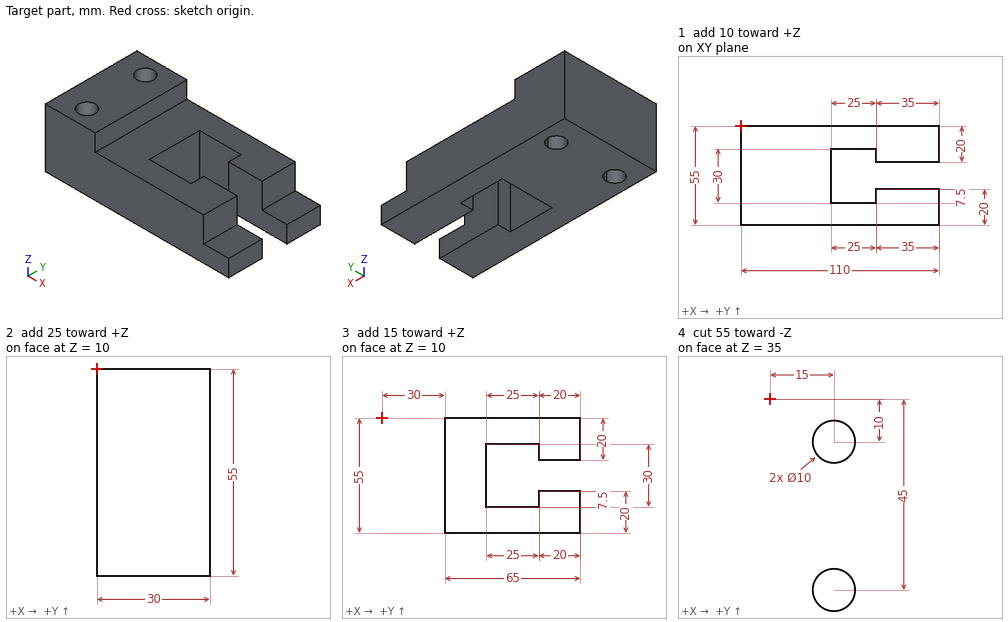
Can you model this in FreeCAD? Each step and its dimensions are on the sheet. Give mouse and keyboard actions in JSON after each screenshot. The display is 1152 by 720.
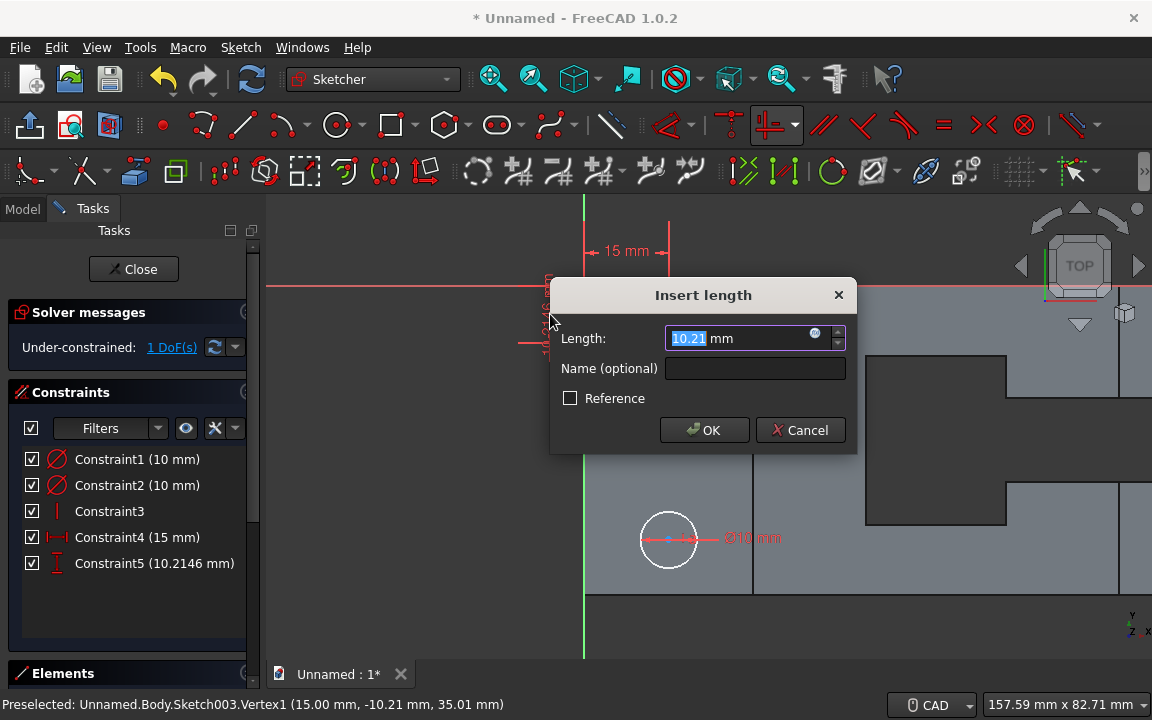
{"action": "type", "text": "10"}
{"action": "key", "text": "Return"}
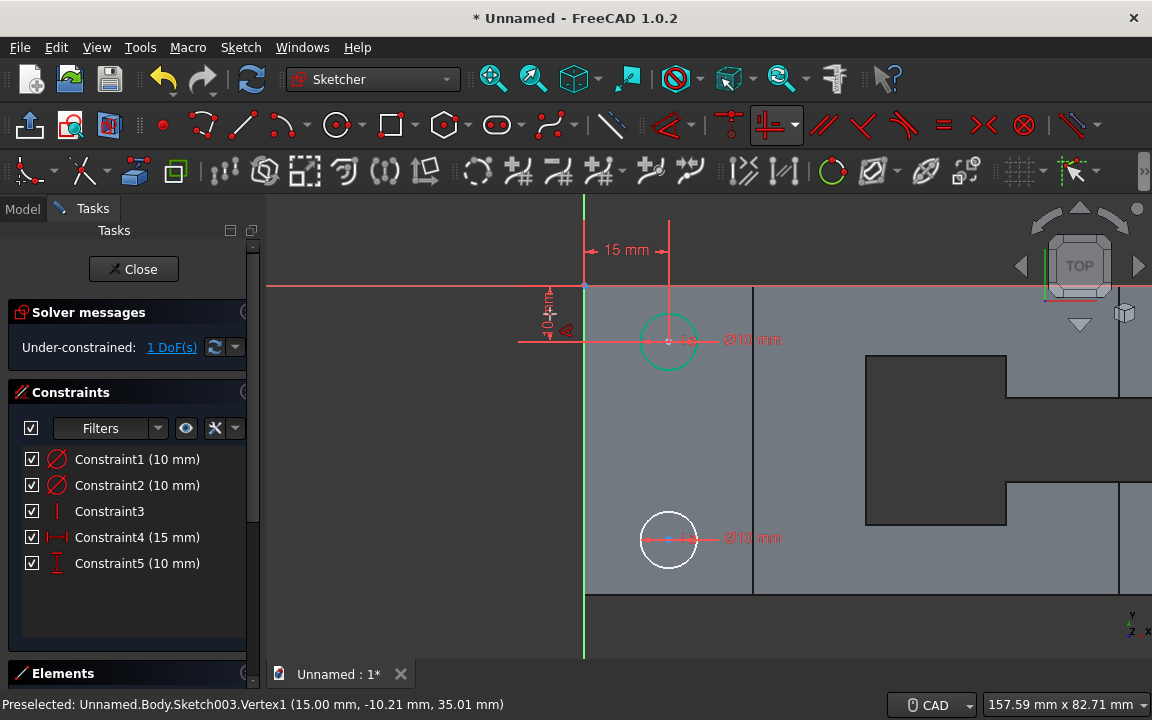
{"action": "left_click", "coordinate": [669, 540]}
{"action": "left_click", "coordinate": [550, 413]}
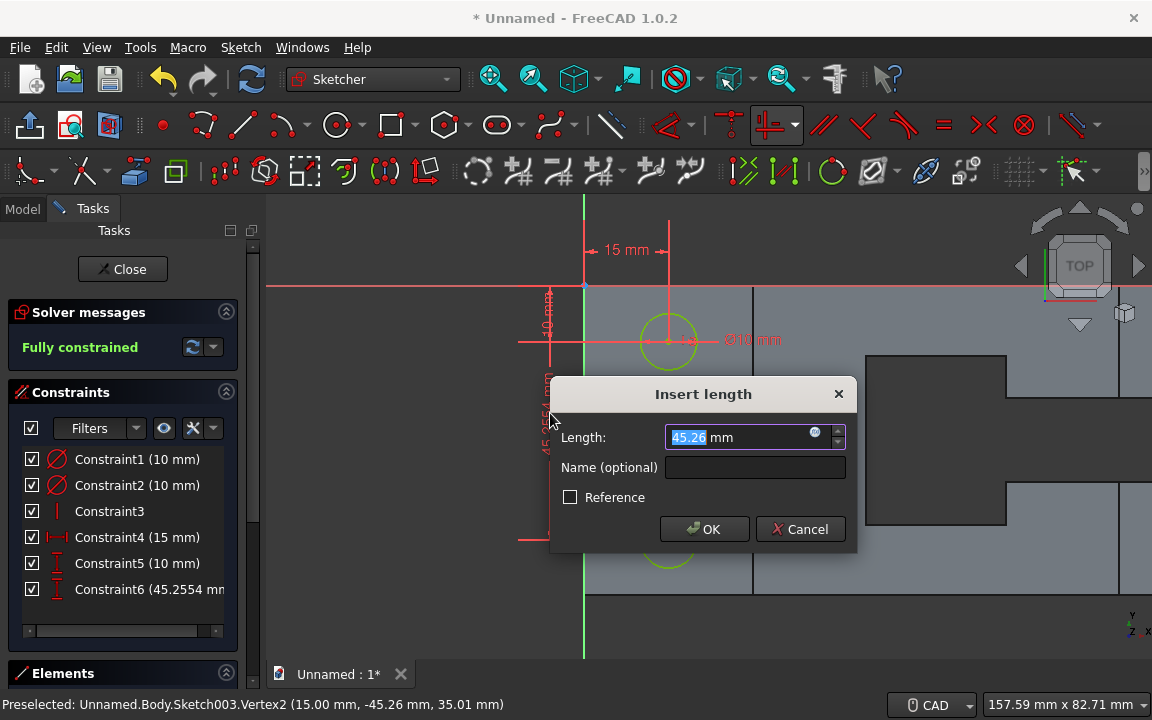
{"action": "type", "text": "45"}
{"action": "key", "text": "Return"}
{"action": "key", "text": "Escape"}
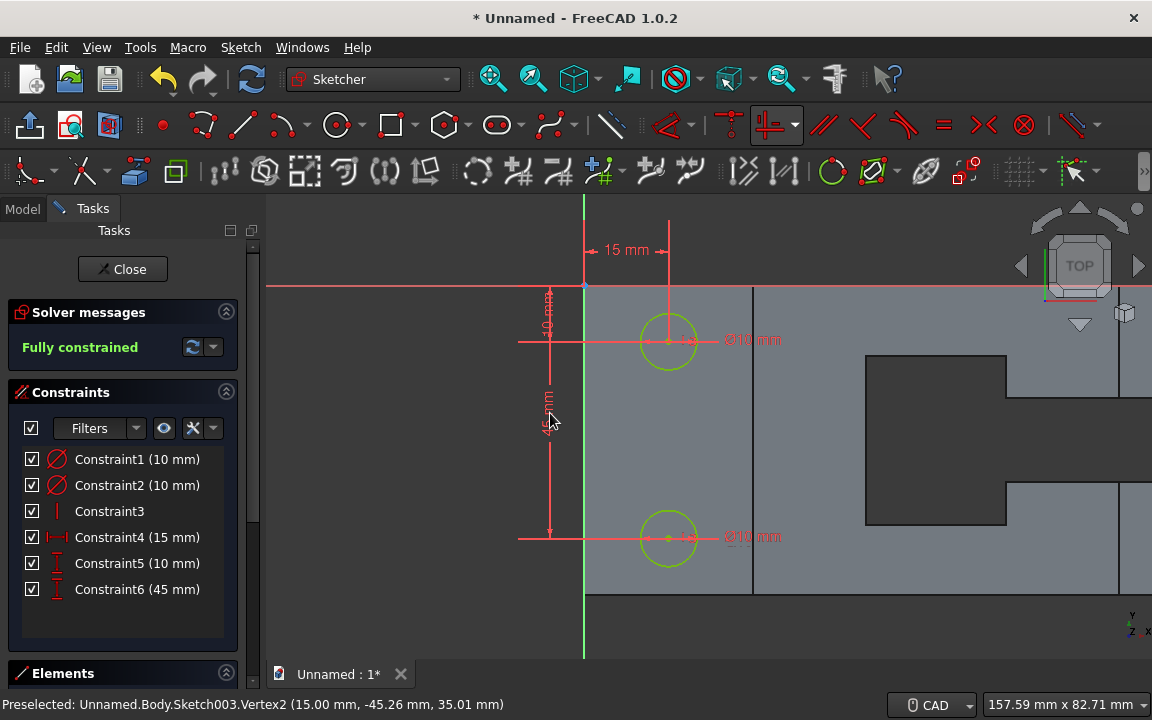
{"action": "left_click", "coordinate": [123, 269]}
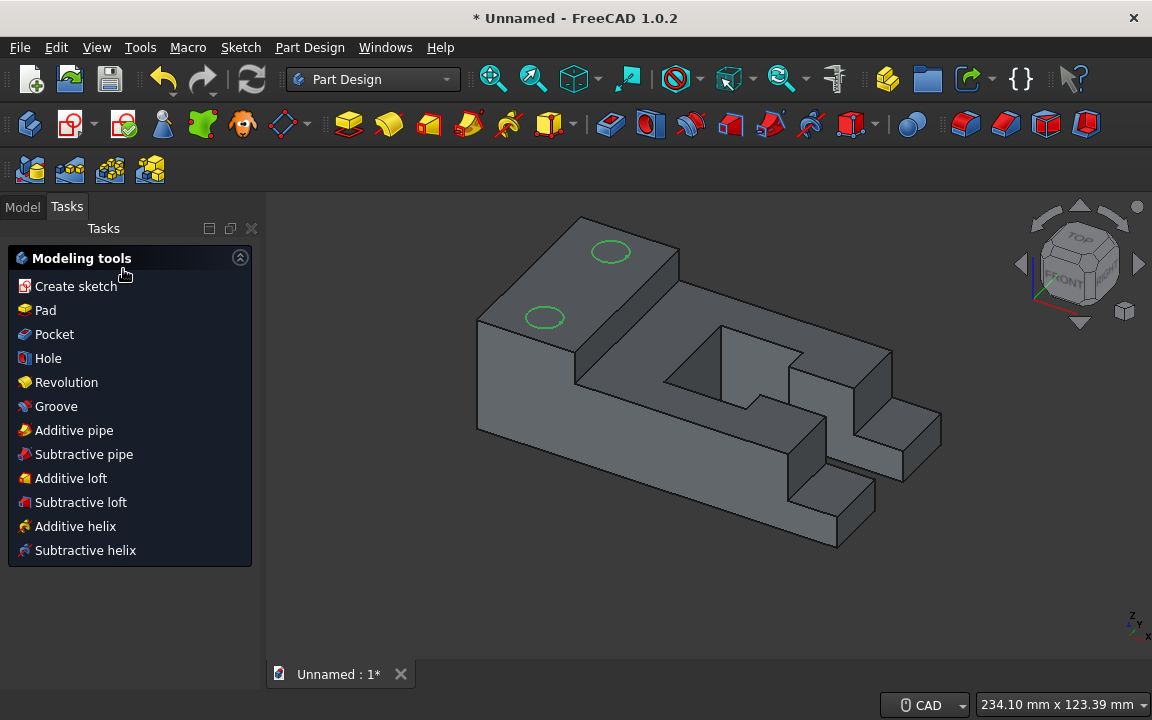
{"action": "left_click", "coordinate": [612, 124]}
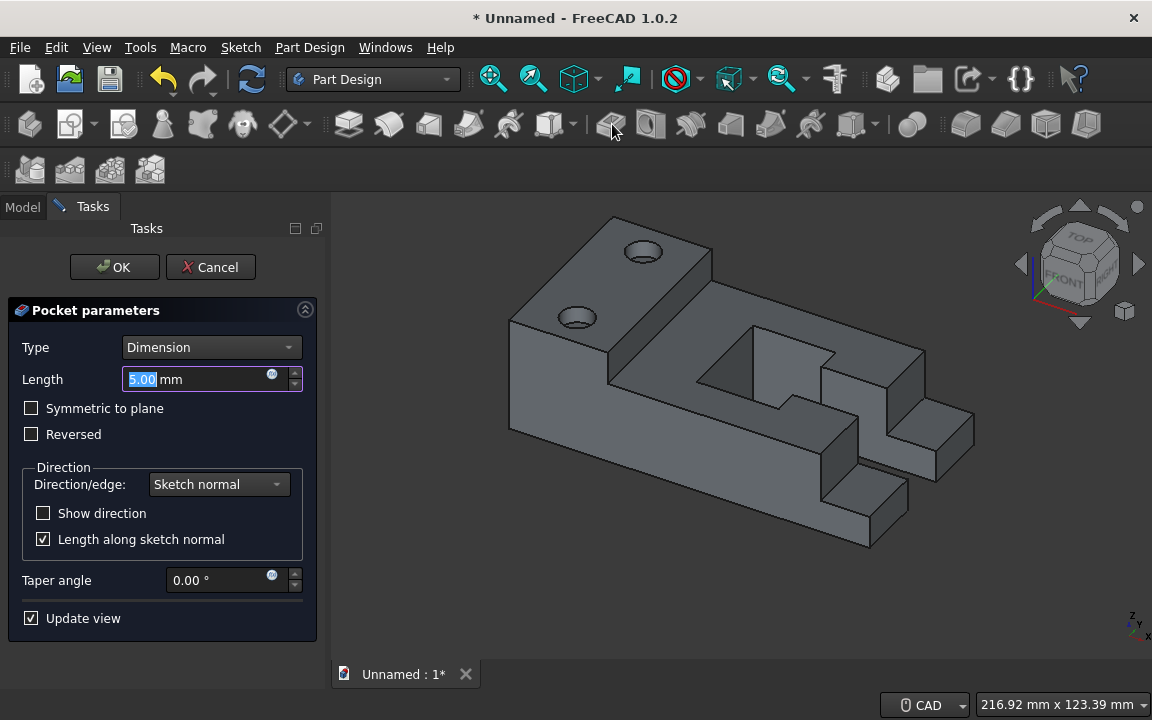
{"action": "type", "text": "55"}
{"action": "key", "text": "Tab"}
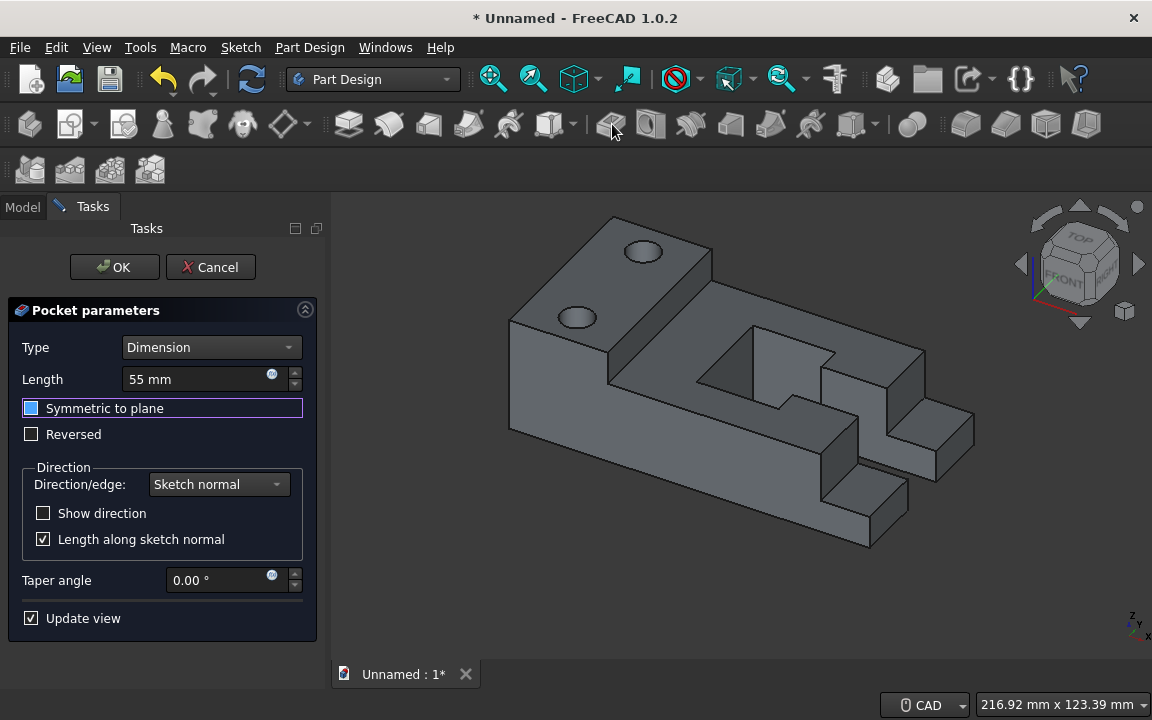
{"action": "left_click", "coordinate": [115, 267]}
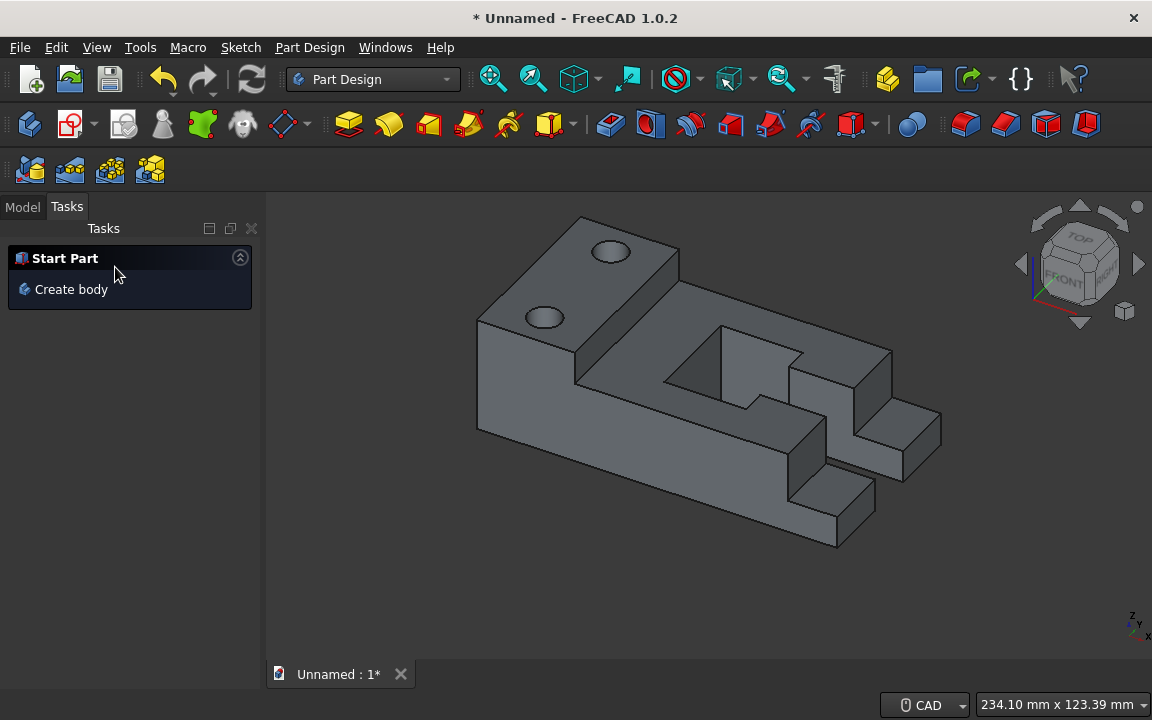
{"action": "key", "text": "0"}